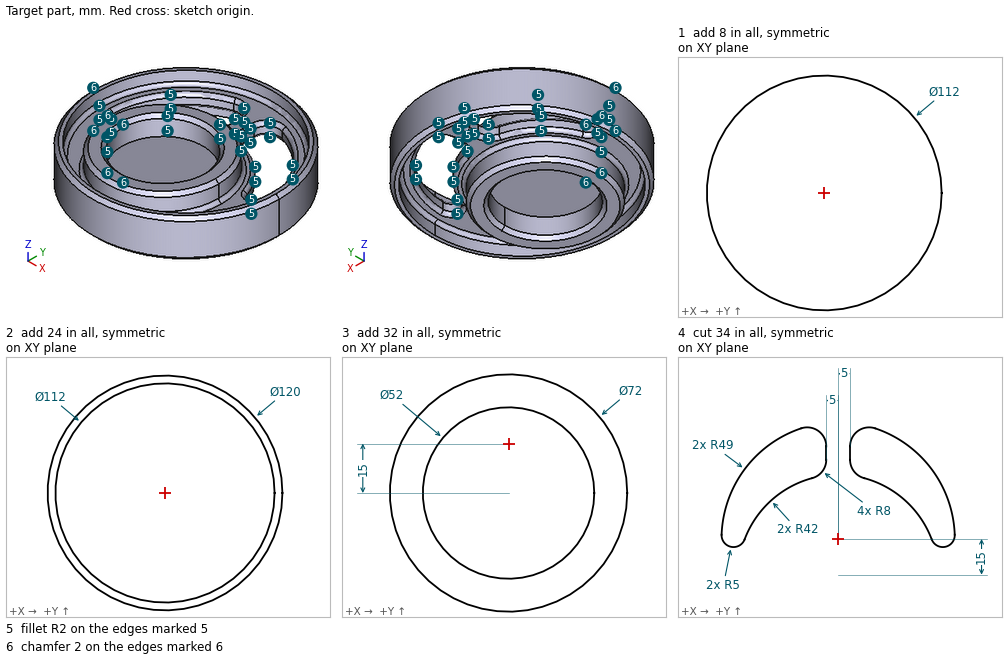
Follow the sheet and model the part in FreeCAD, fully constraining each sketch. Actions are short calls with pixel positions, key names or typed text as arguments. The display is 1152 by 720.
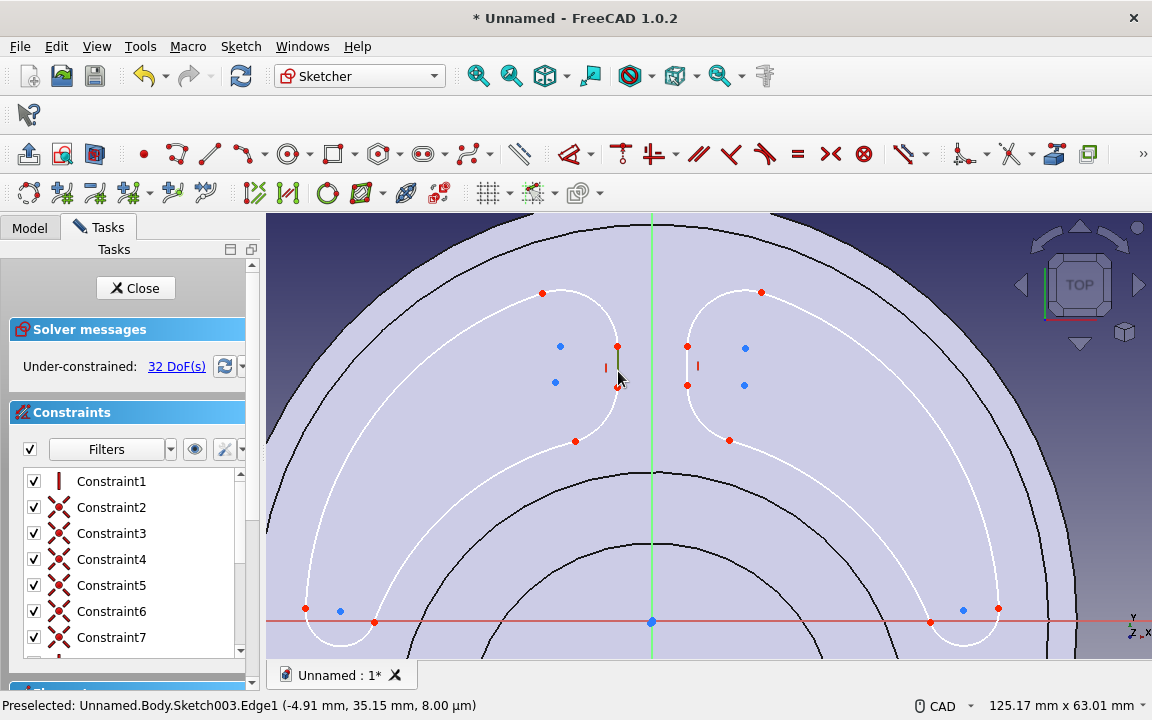
click(609, 316)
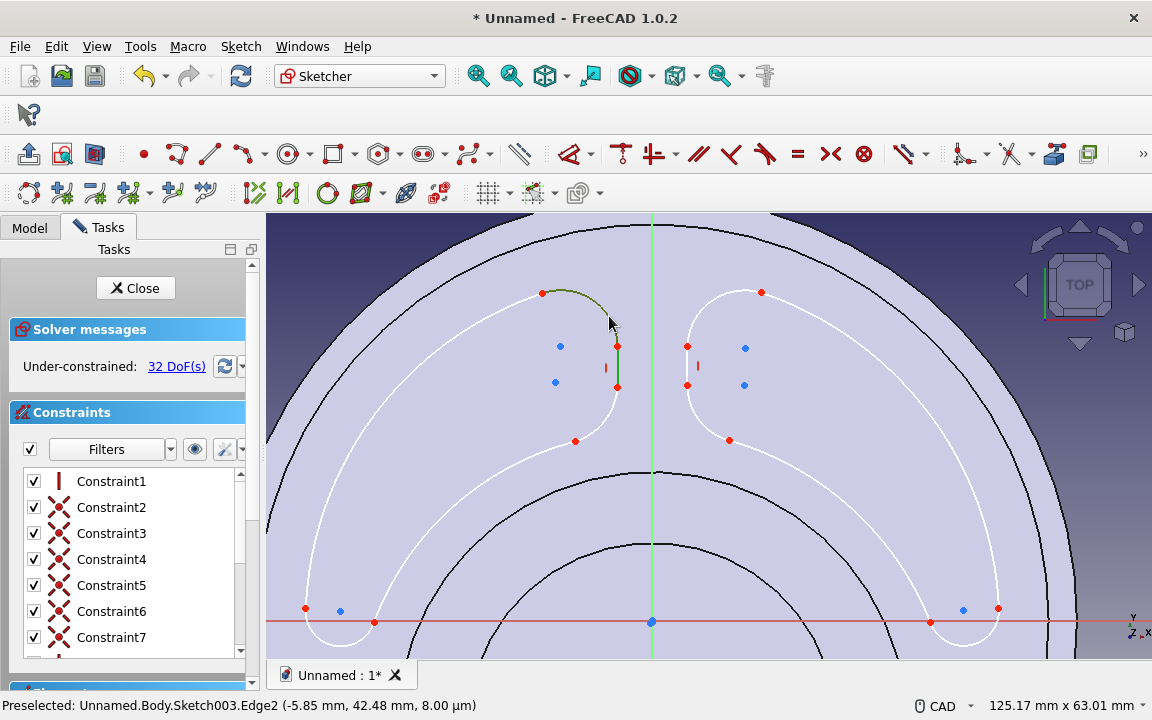
click(765, 154)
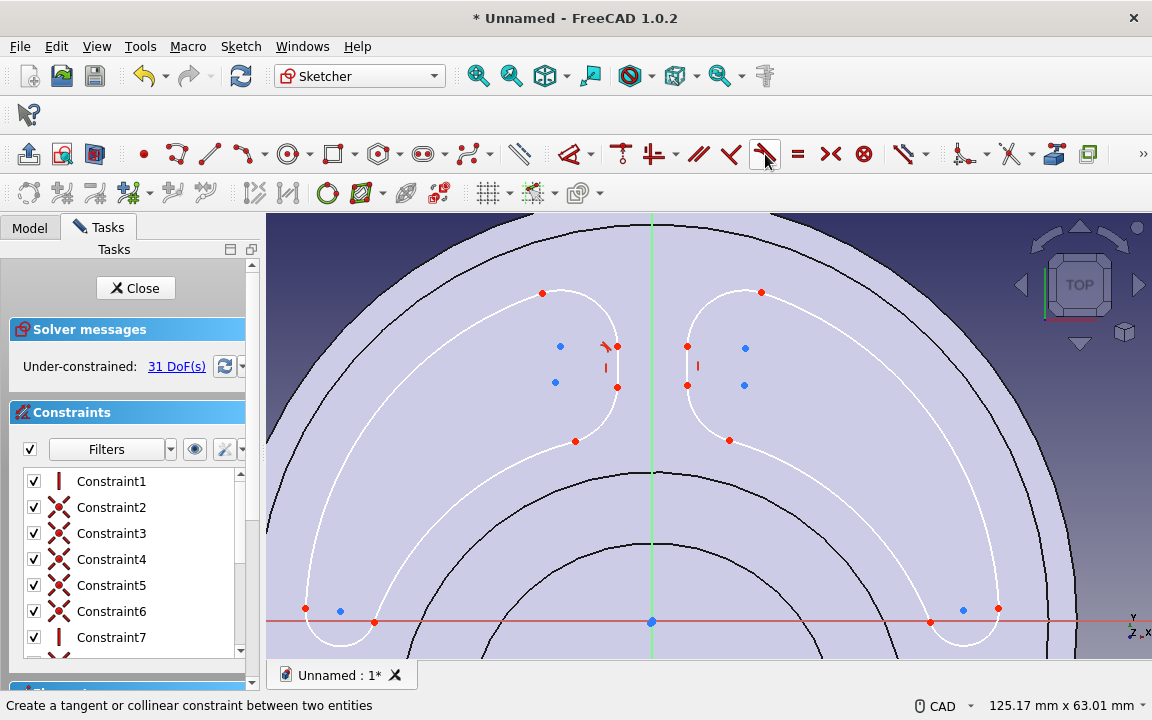
click(618, 375)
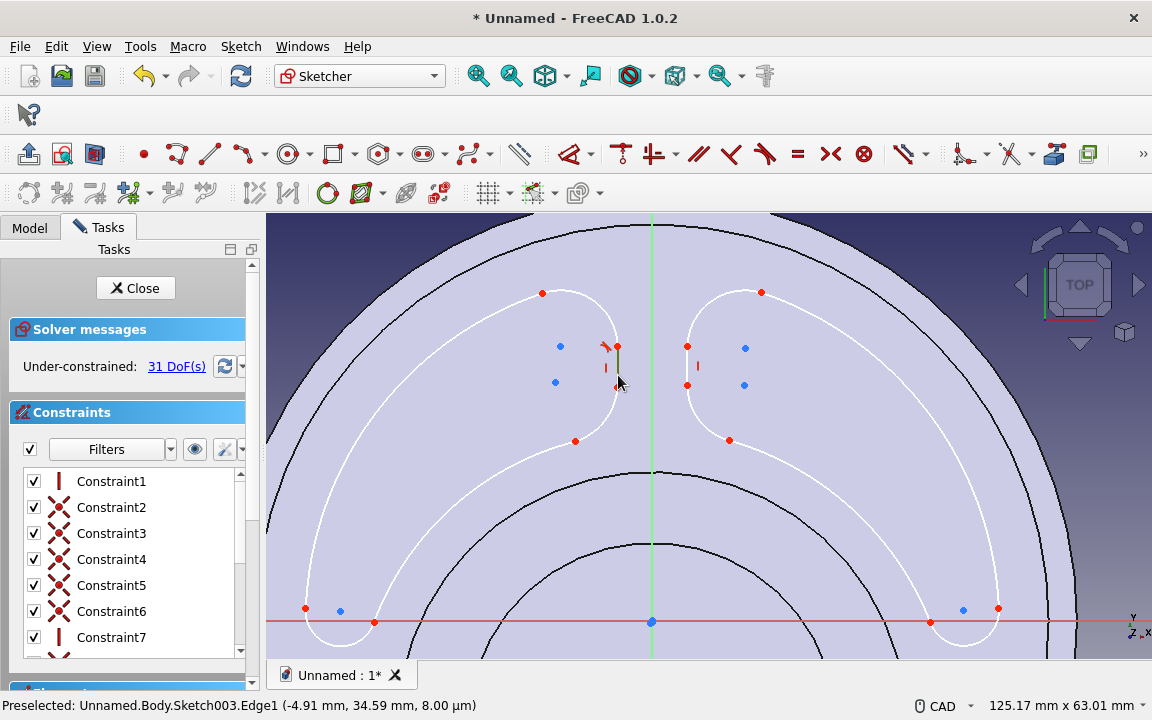
click(595, 431)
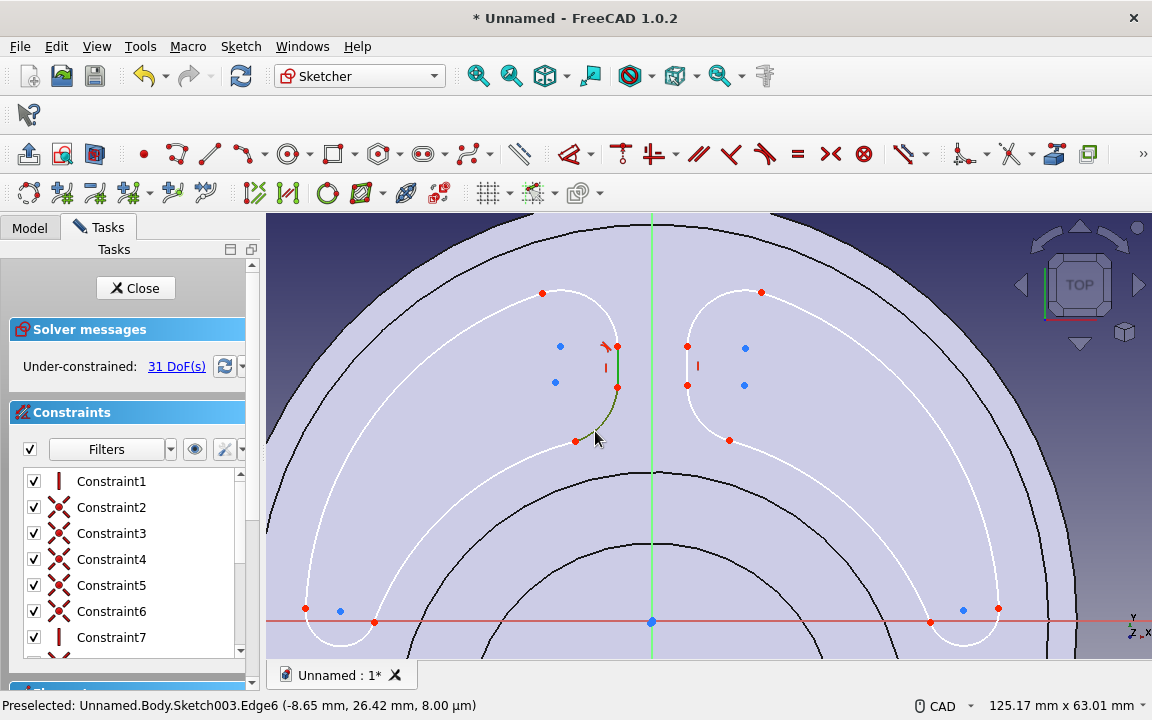
key(t)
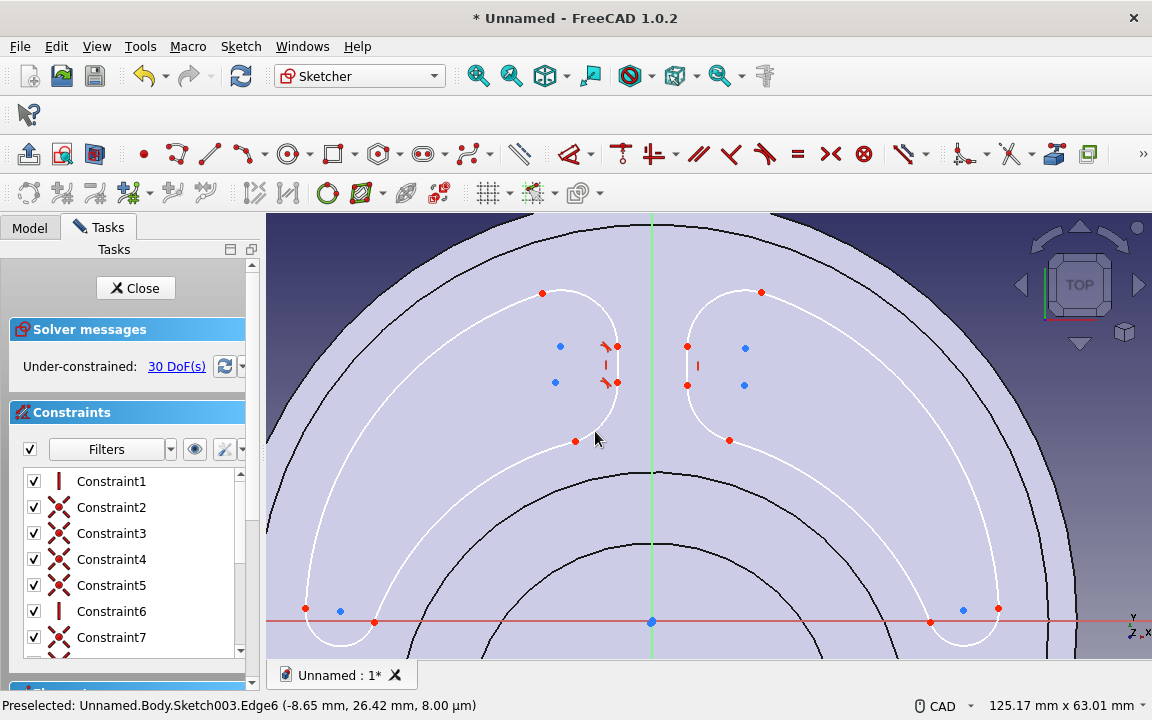
click(609, 316)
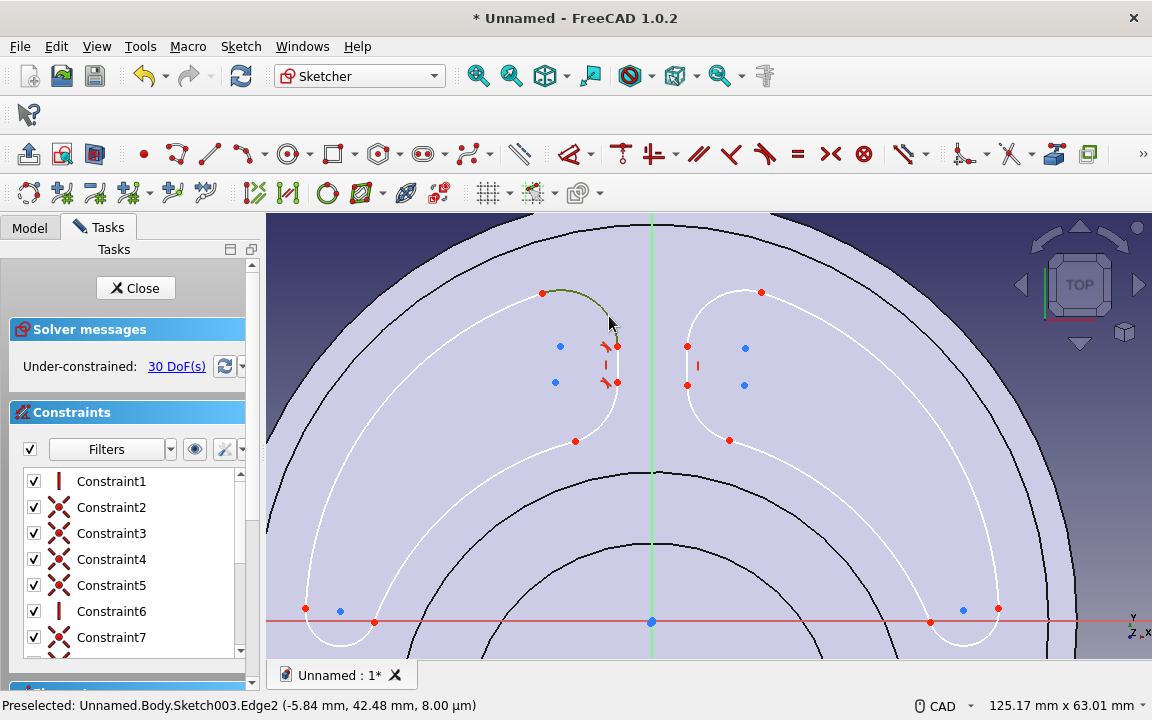
click(433, 354)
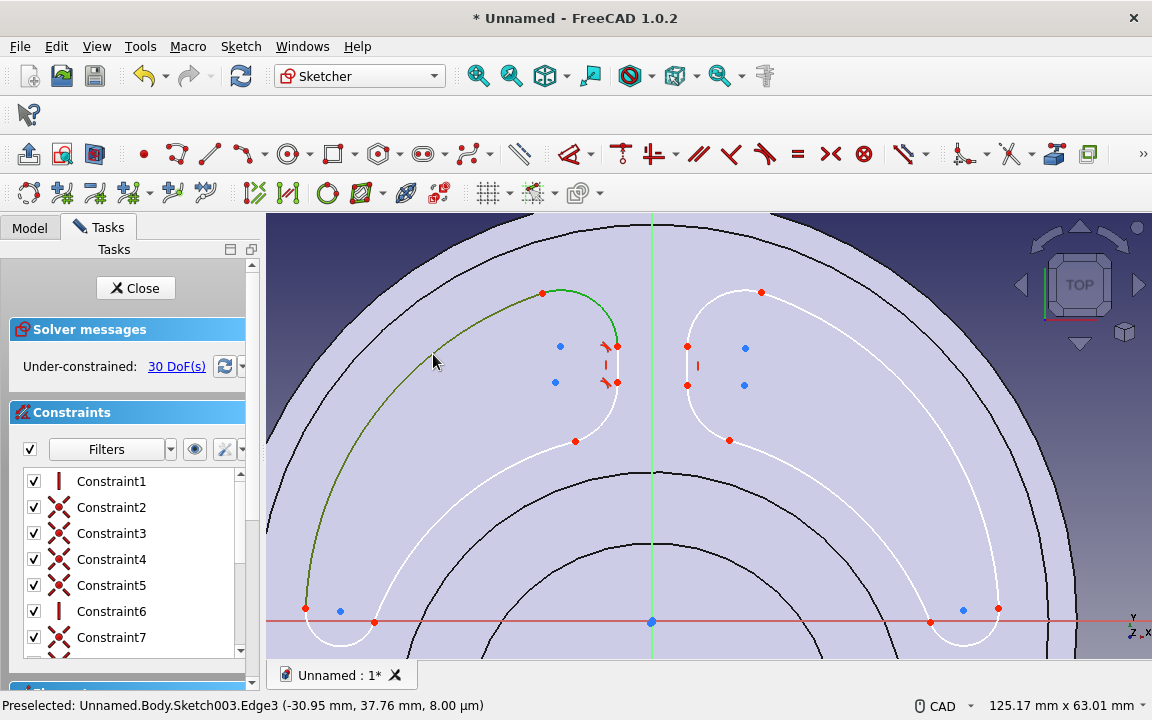
key(t)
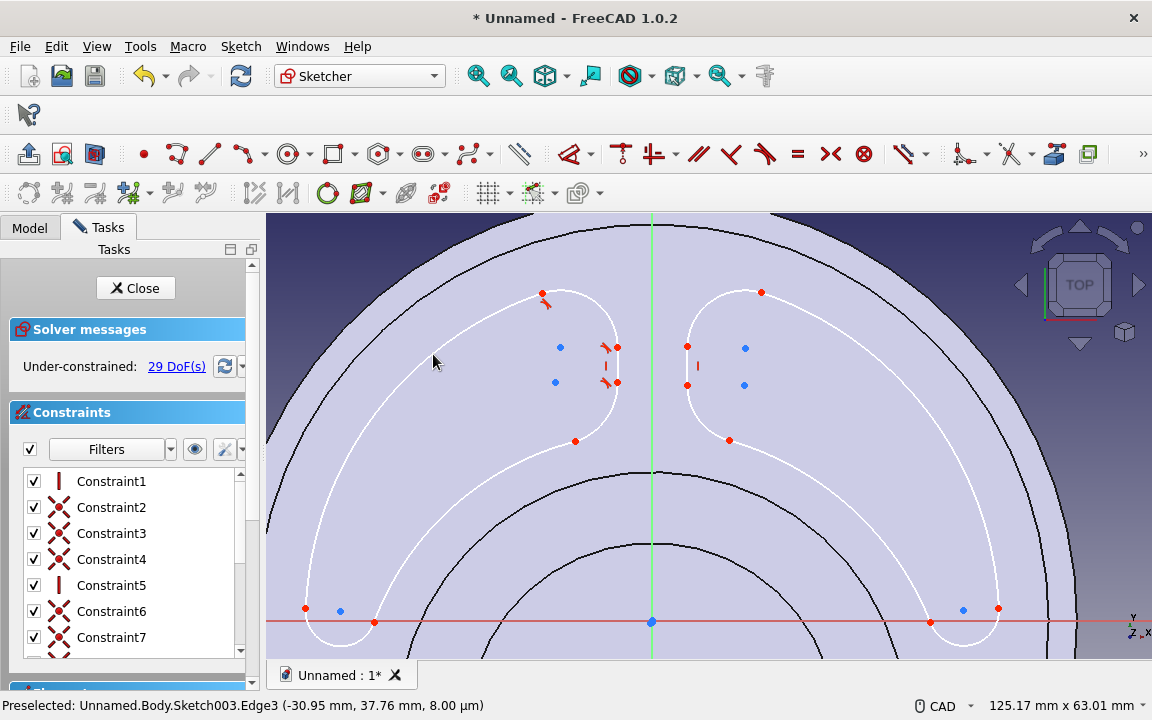
click(433, 354)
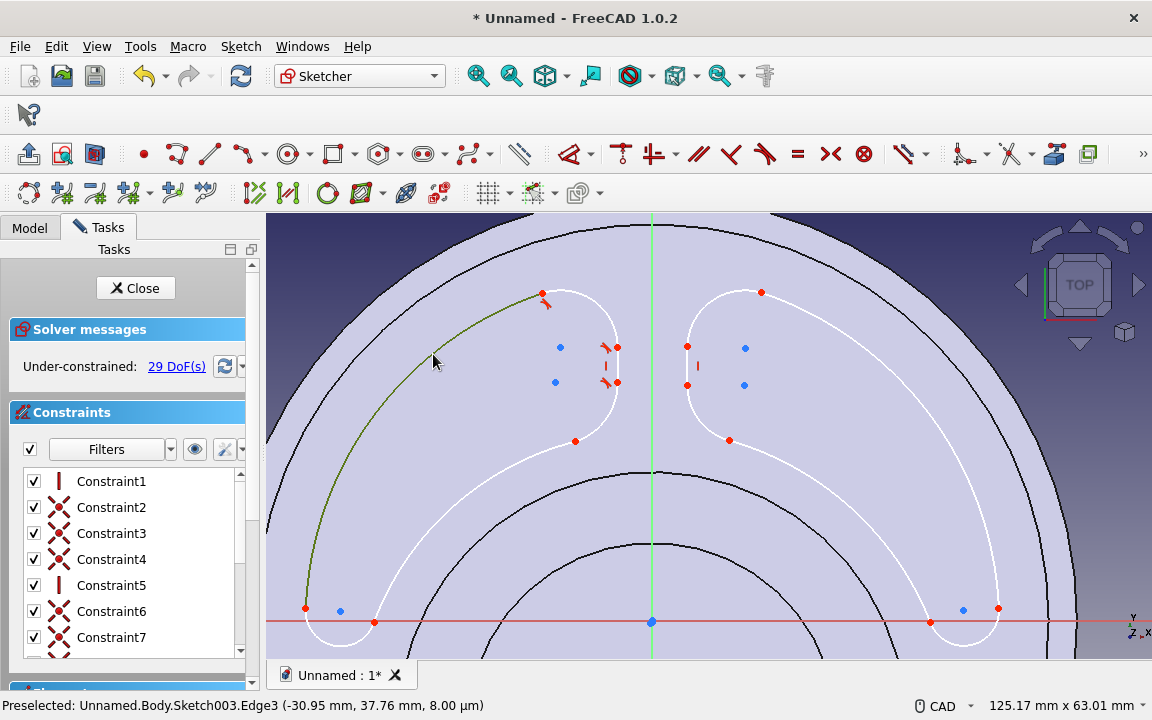
scroll(617, 371, down, 2)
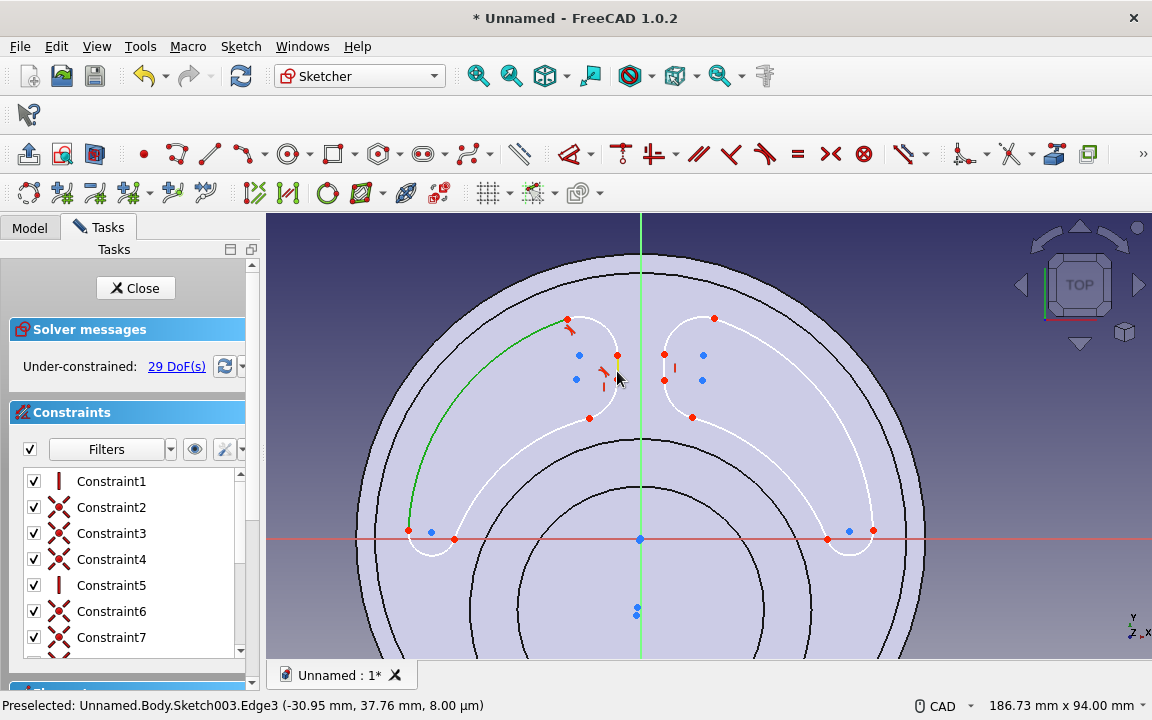
scroll(416, 549, up, 2)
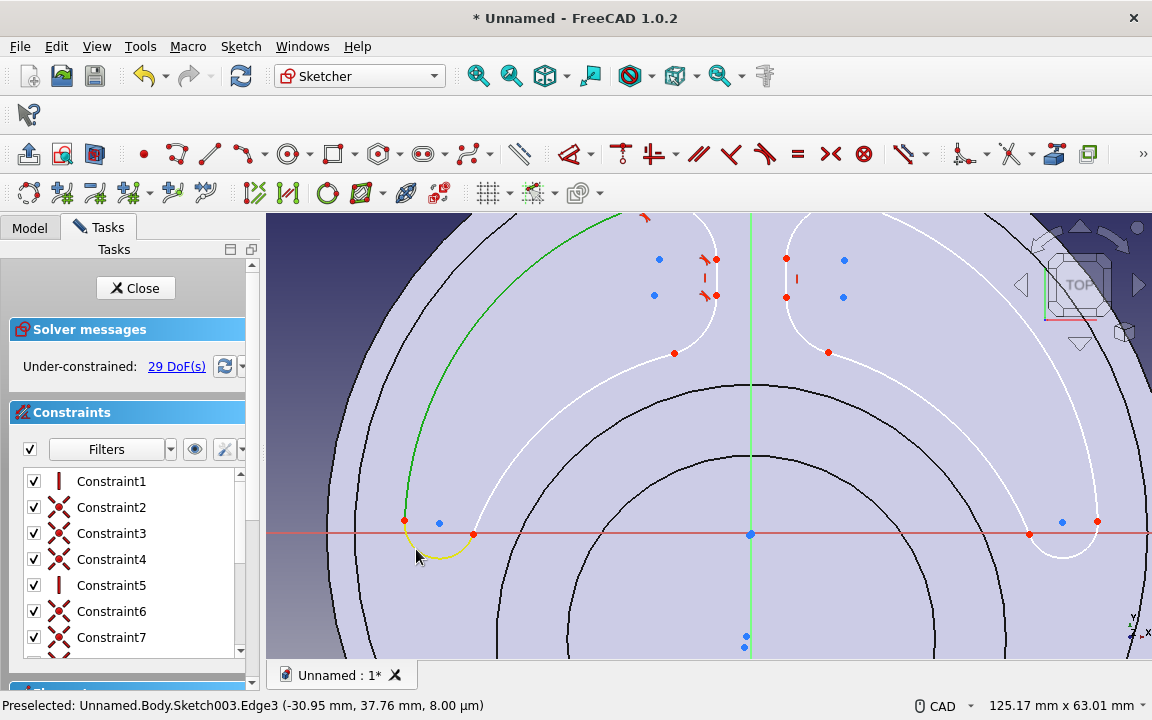
click(415, 549)